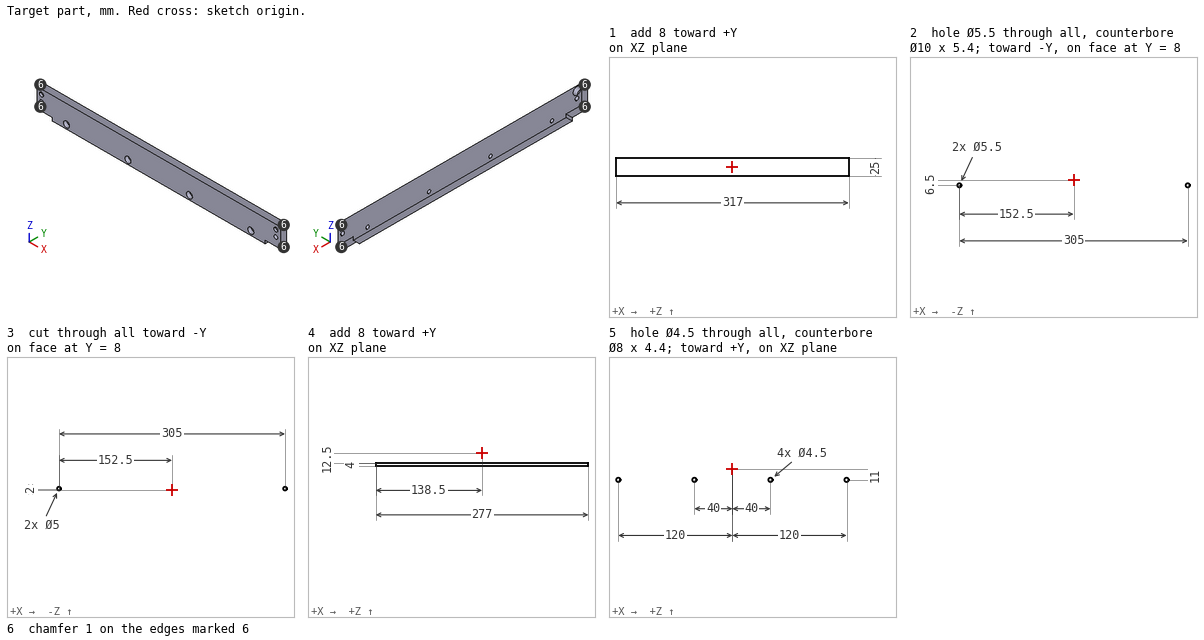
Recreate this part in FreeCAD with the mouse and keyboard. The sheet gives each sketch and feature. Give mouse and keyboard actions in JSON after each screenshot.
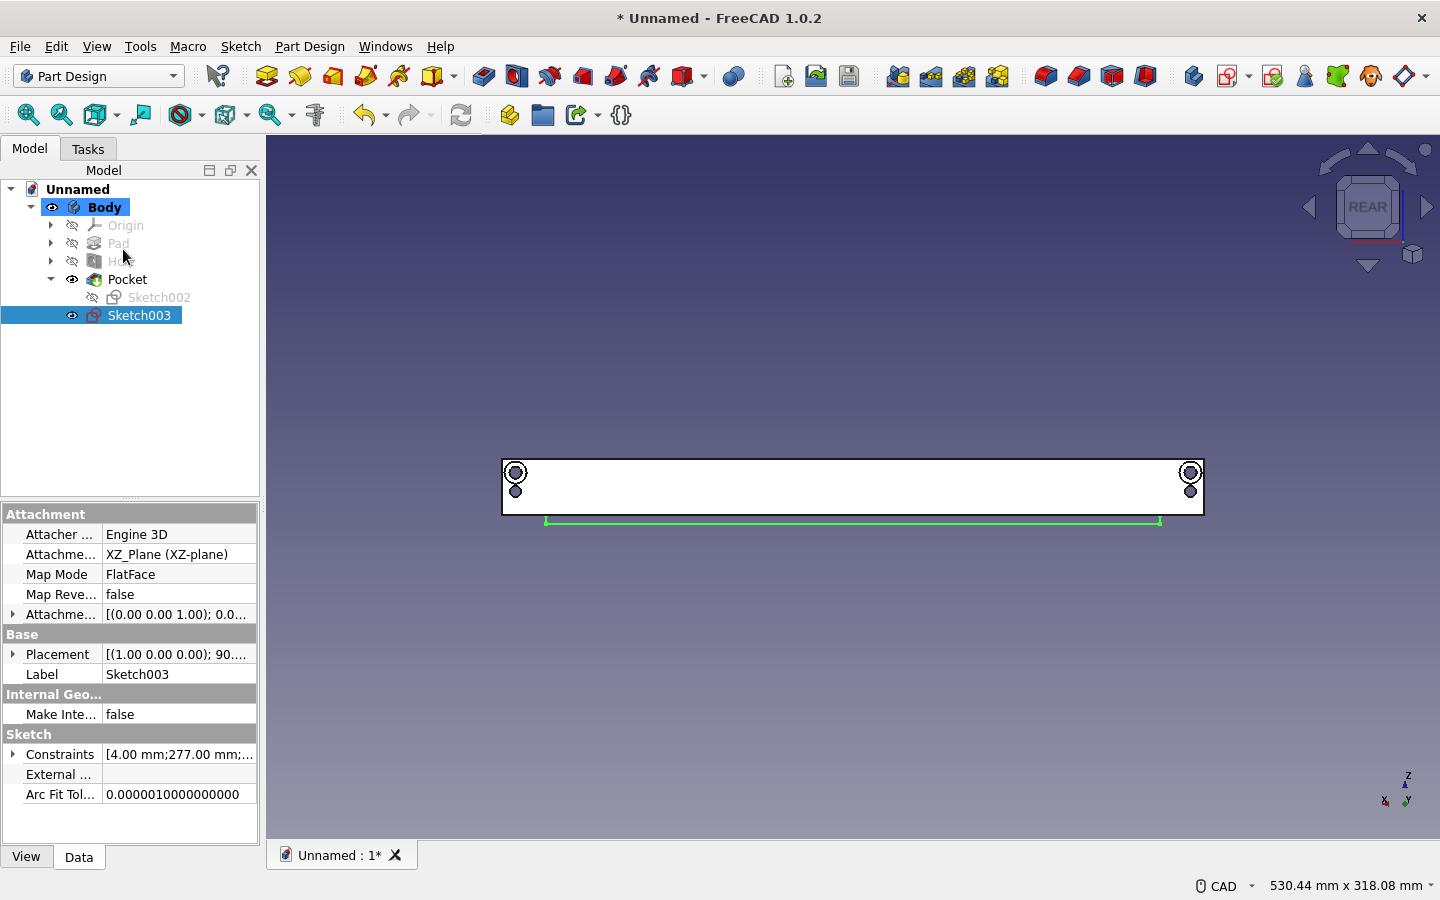
{"action": "left_click", "coordinate": [267, 76]}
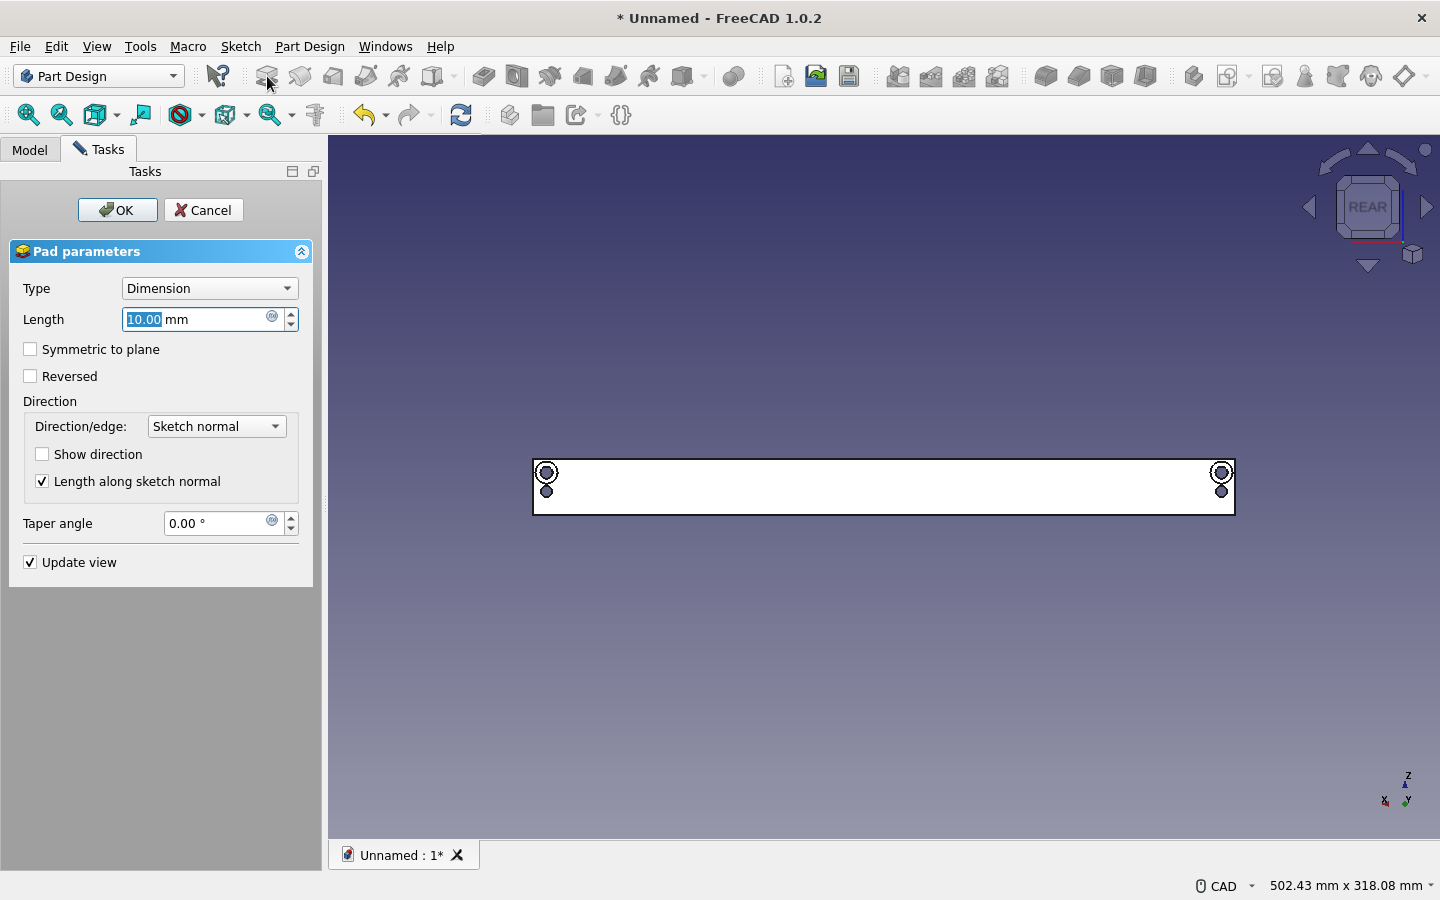
{"action": "type", "text": "8"}
{"action": "key", "text": "Tab"}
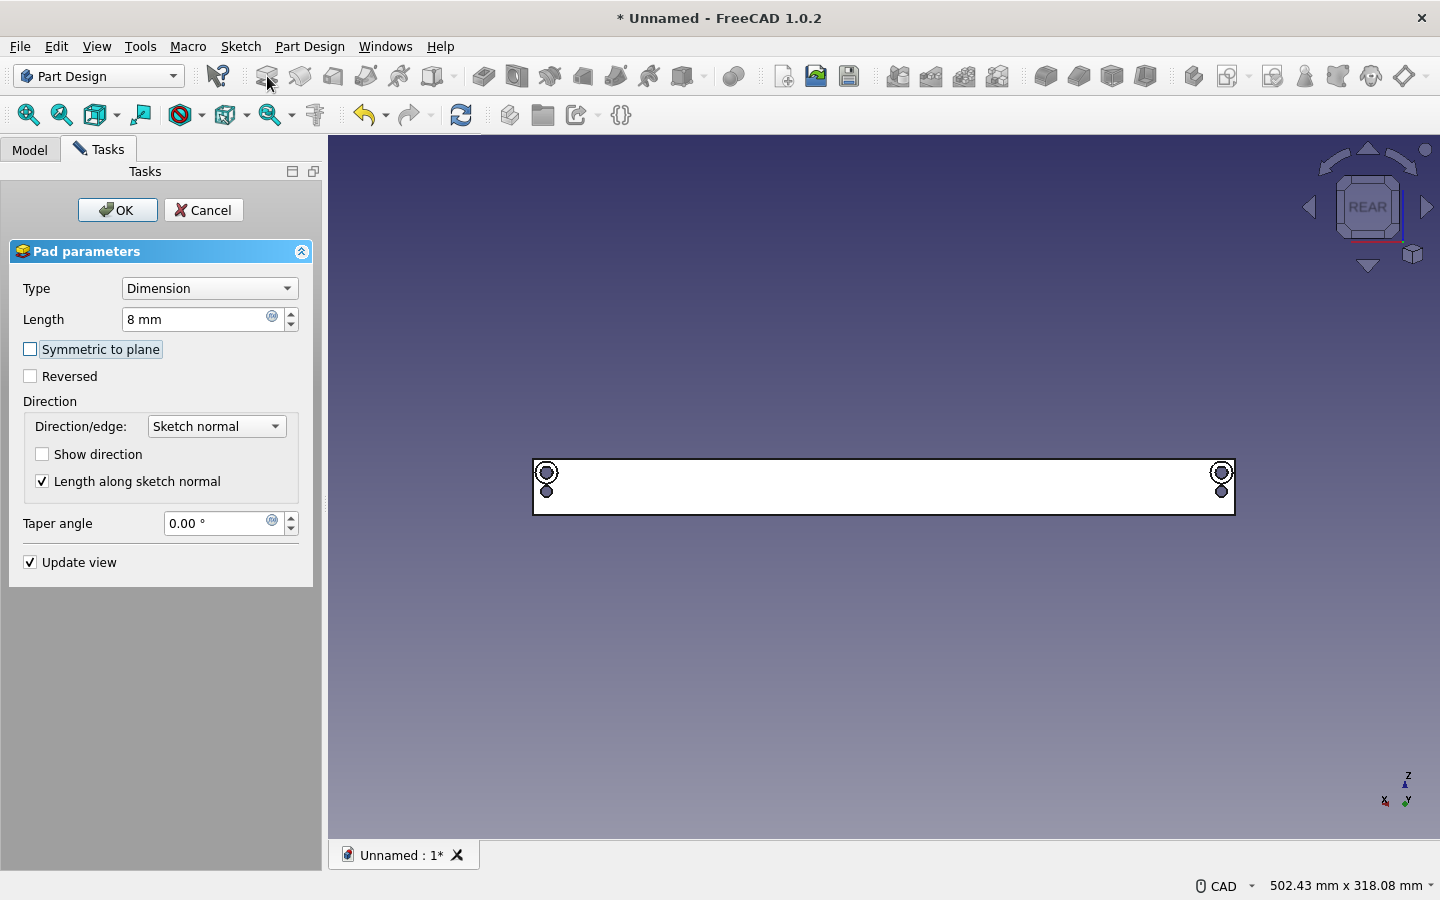
{"action": "left_click", "coordinate": [31, 376]}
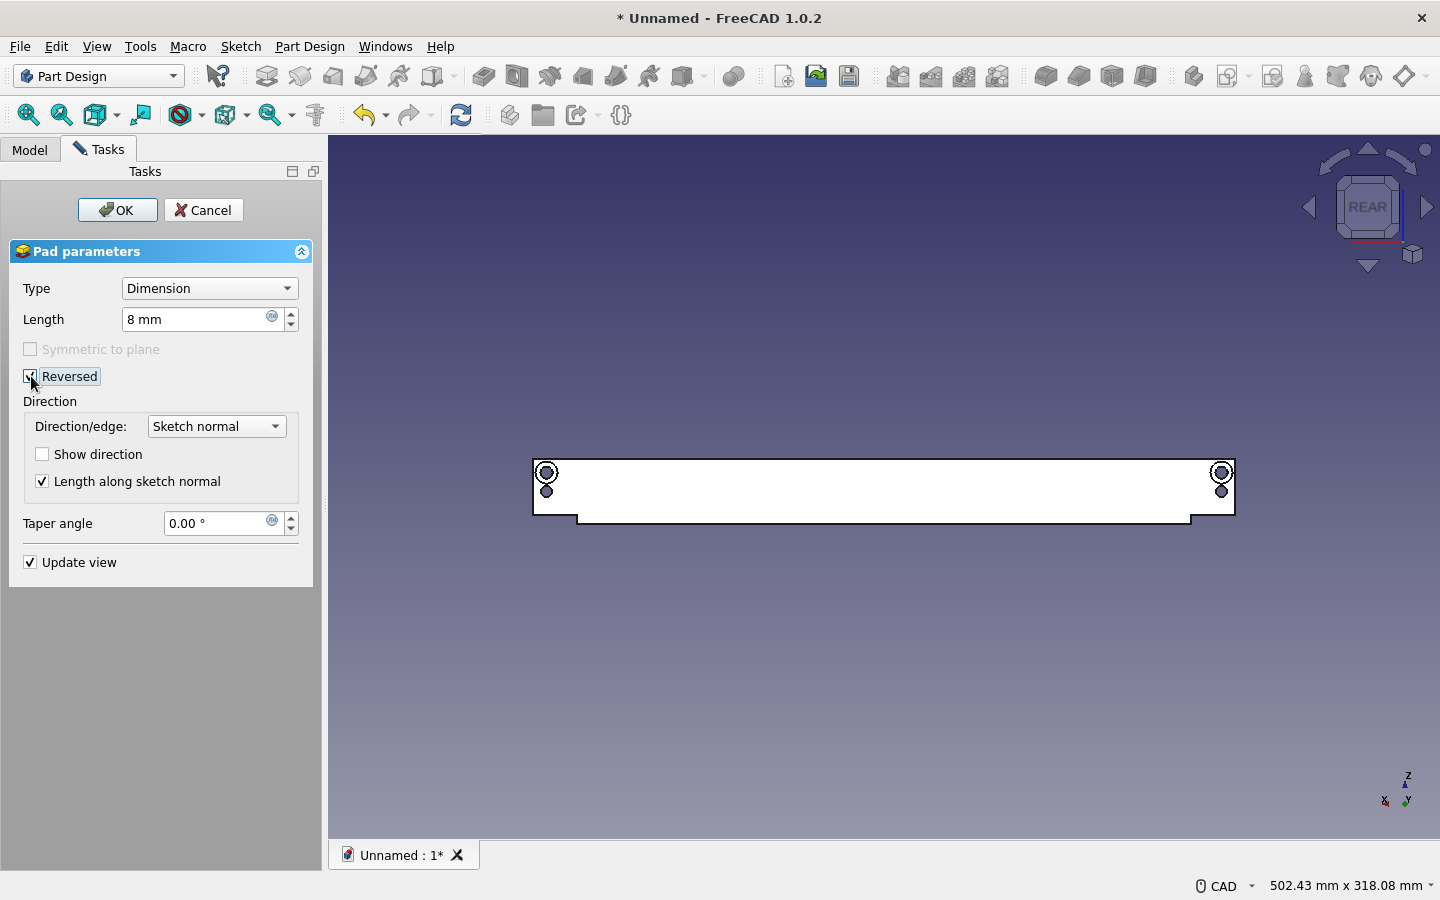
{"action": "left_click", "coordinate": [118, 210]}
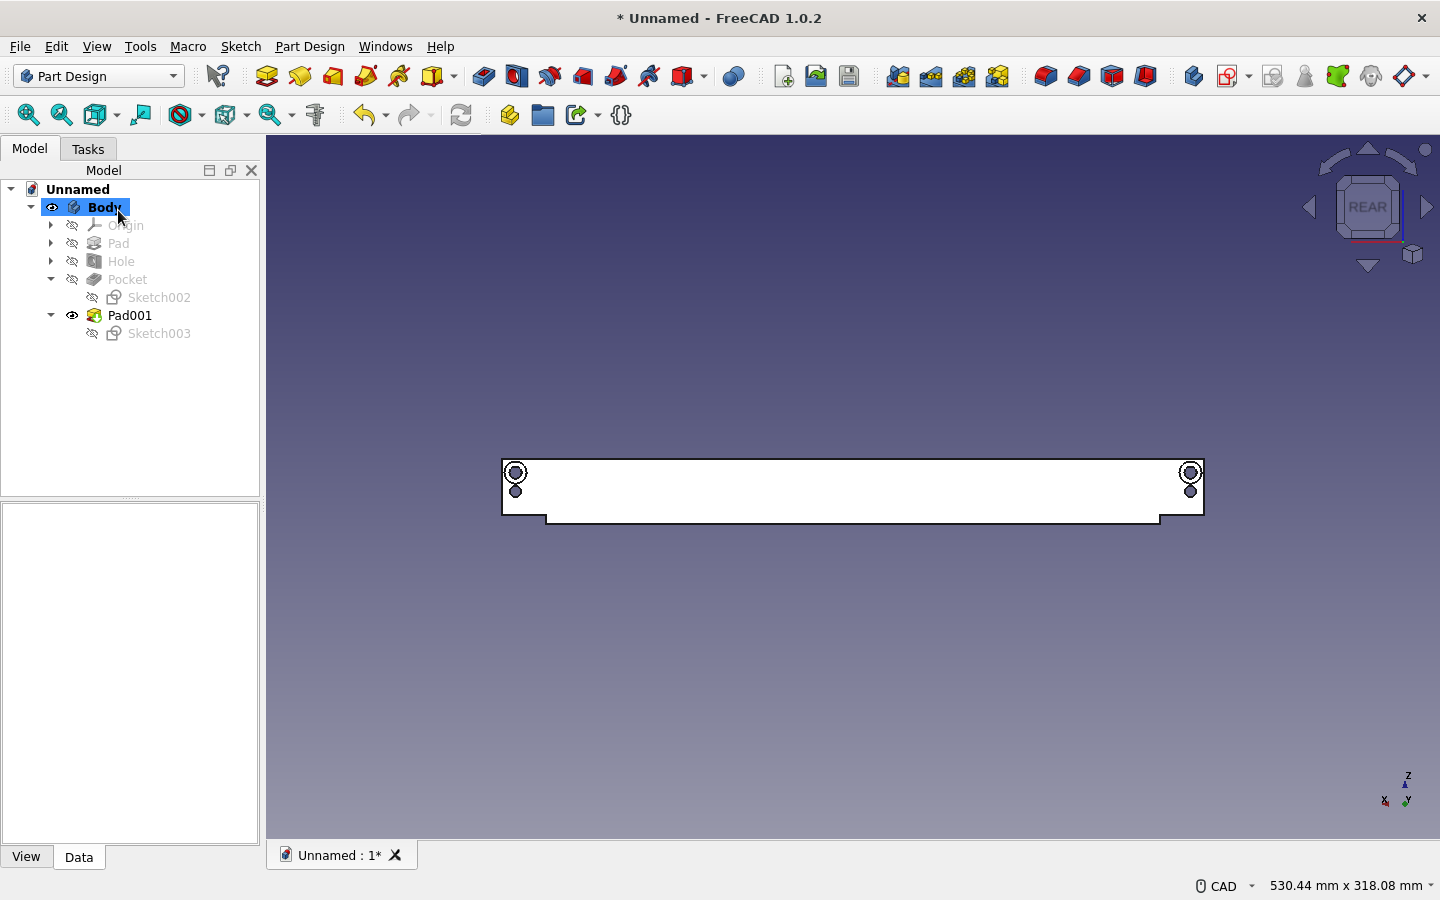
{"action": "left_click", "coordinate": [1226, 76]}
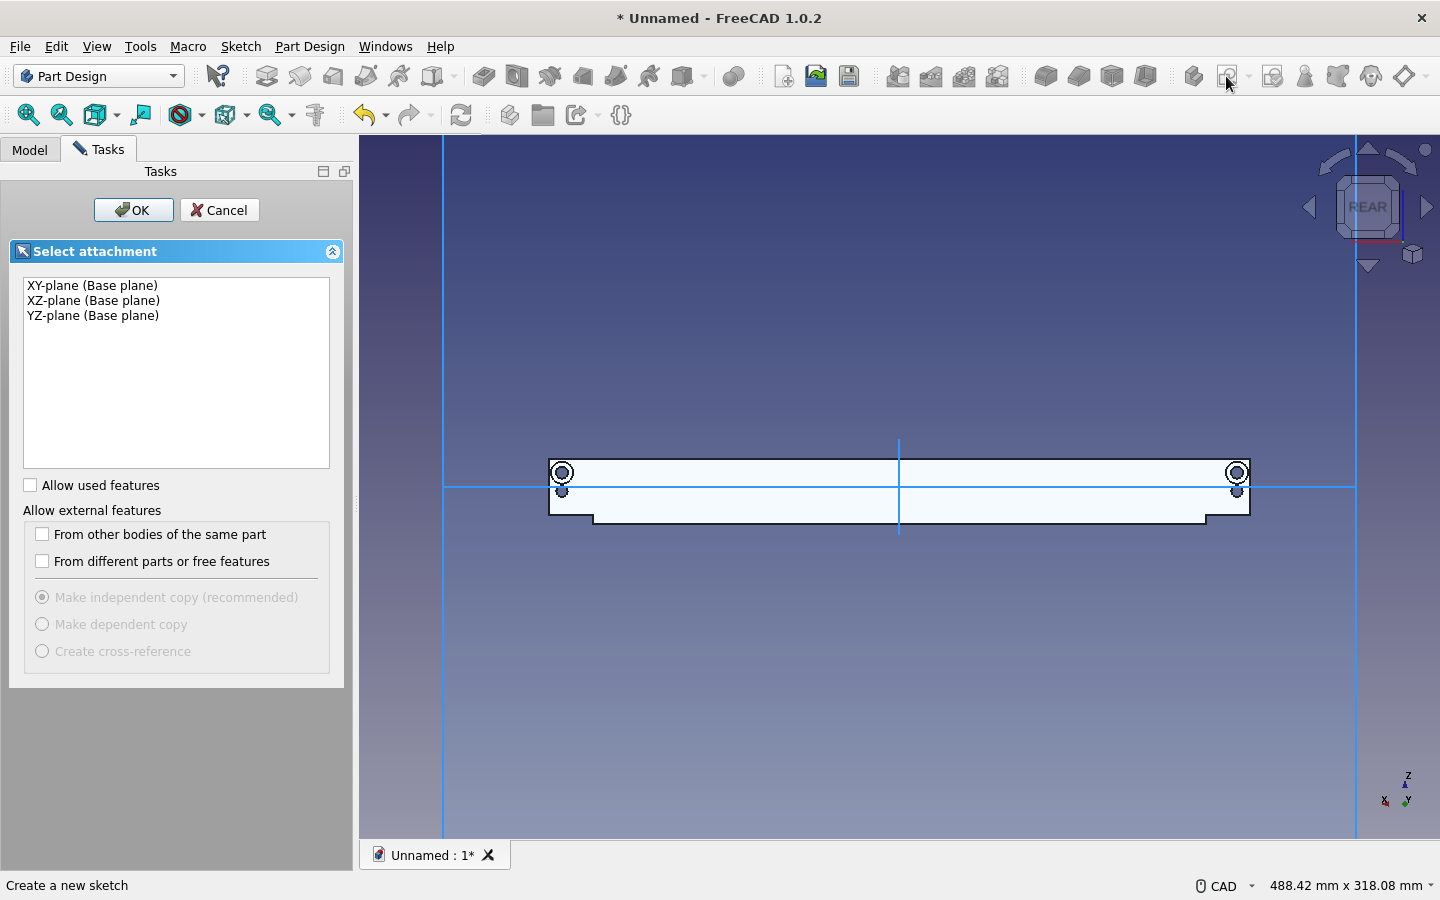
{"action": "left_click", "coordinate": [84, 300]}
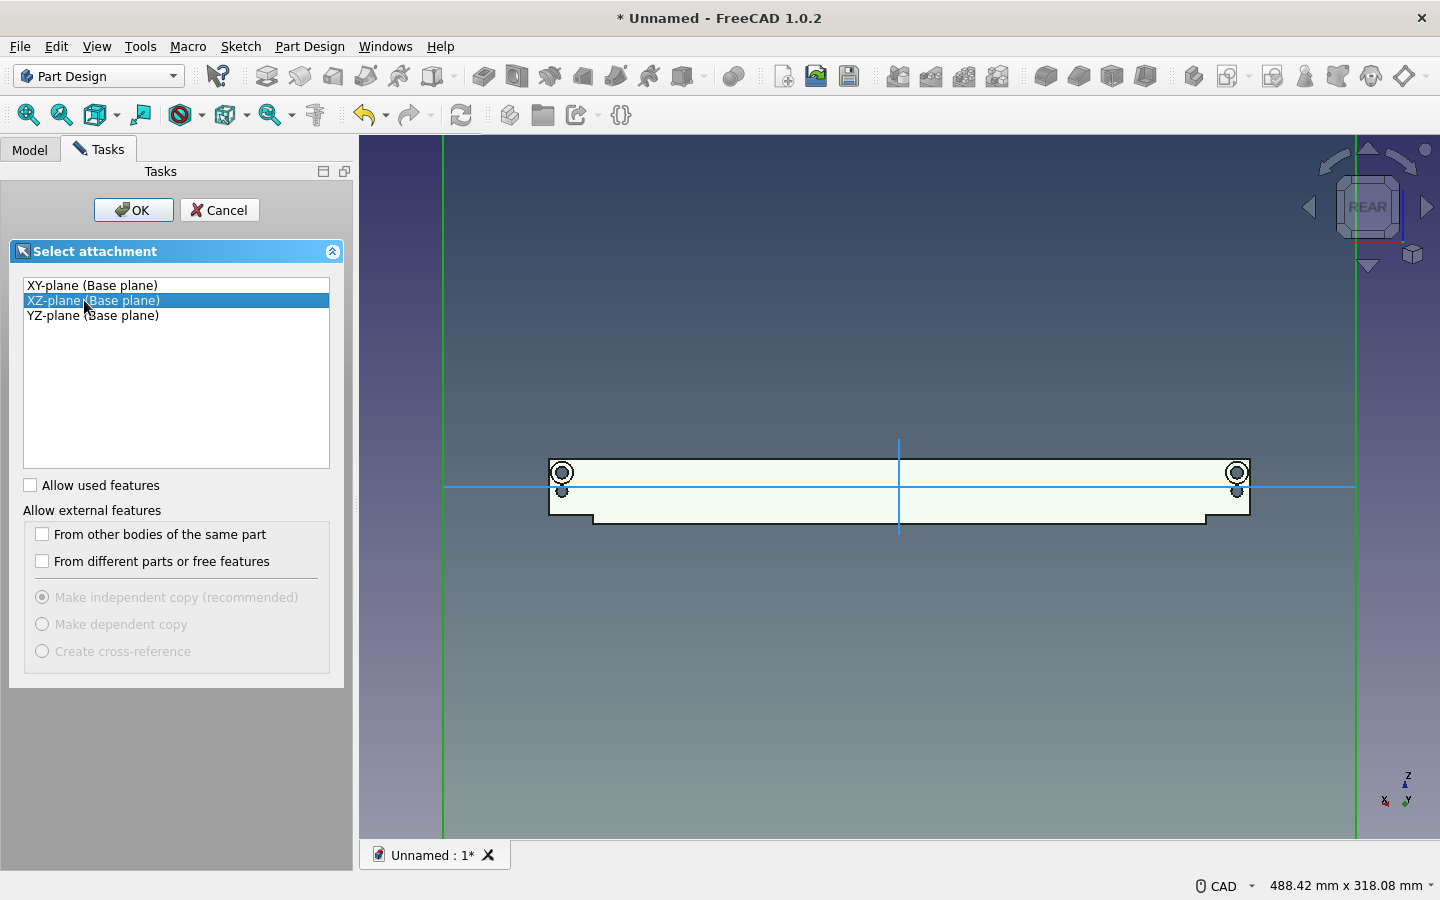
{"action": "left_click", "coordinate": [134, 210]}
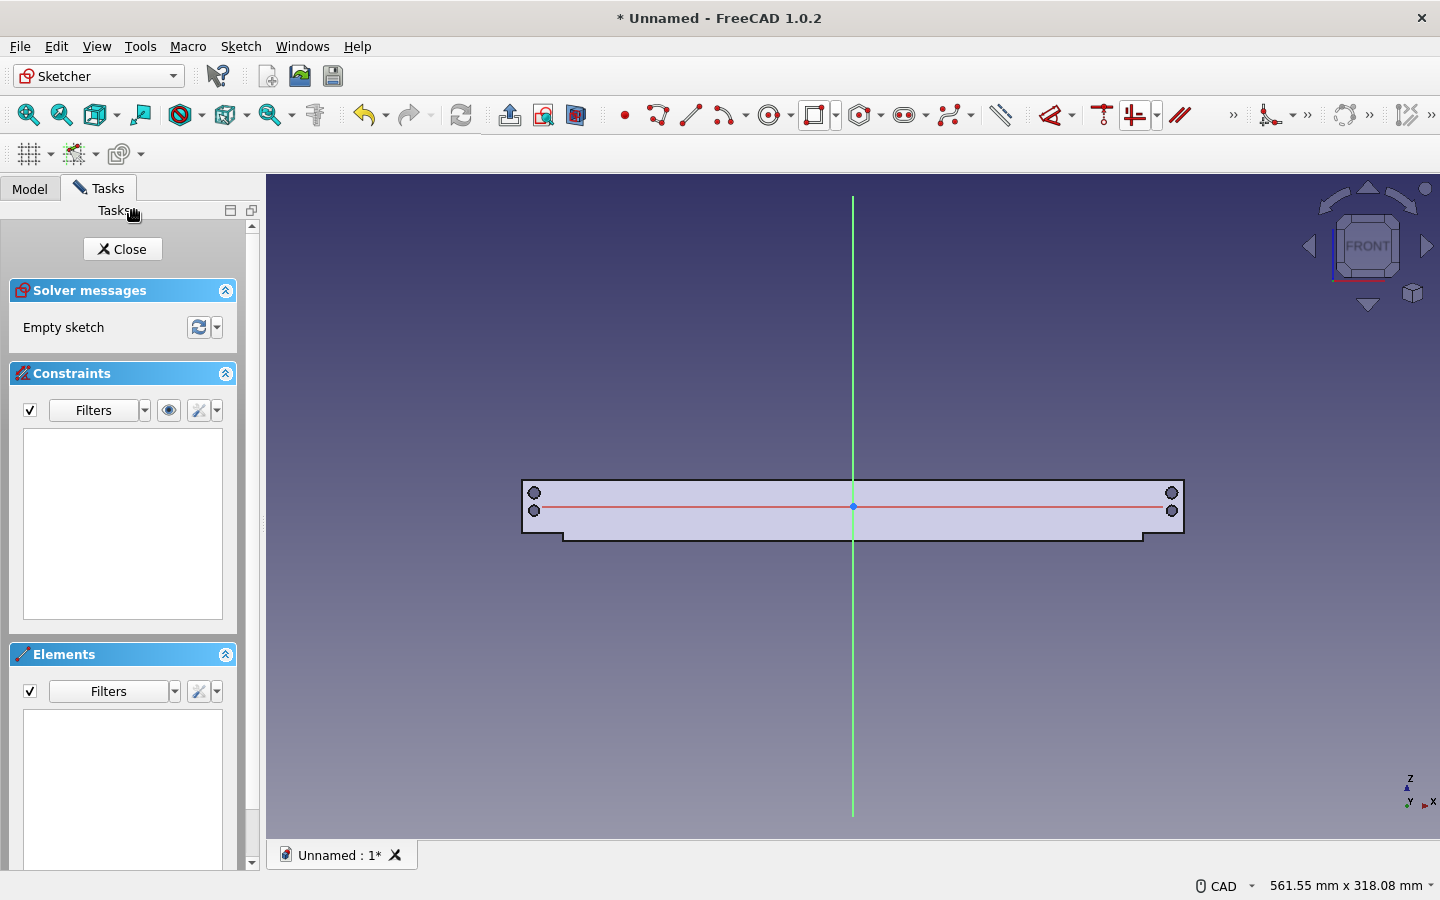
{"action": "scroll", "coordinate": [992, 549], "scroll_direction": "up", "scroll_amount": 2}